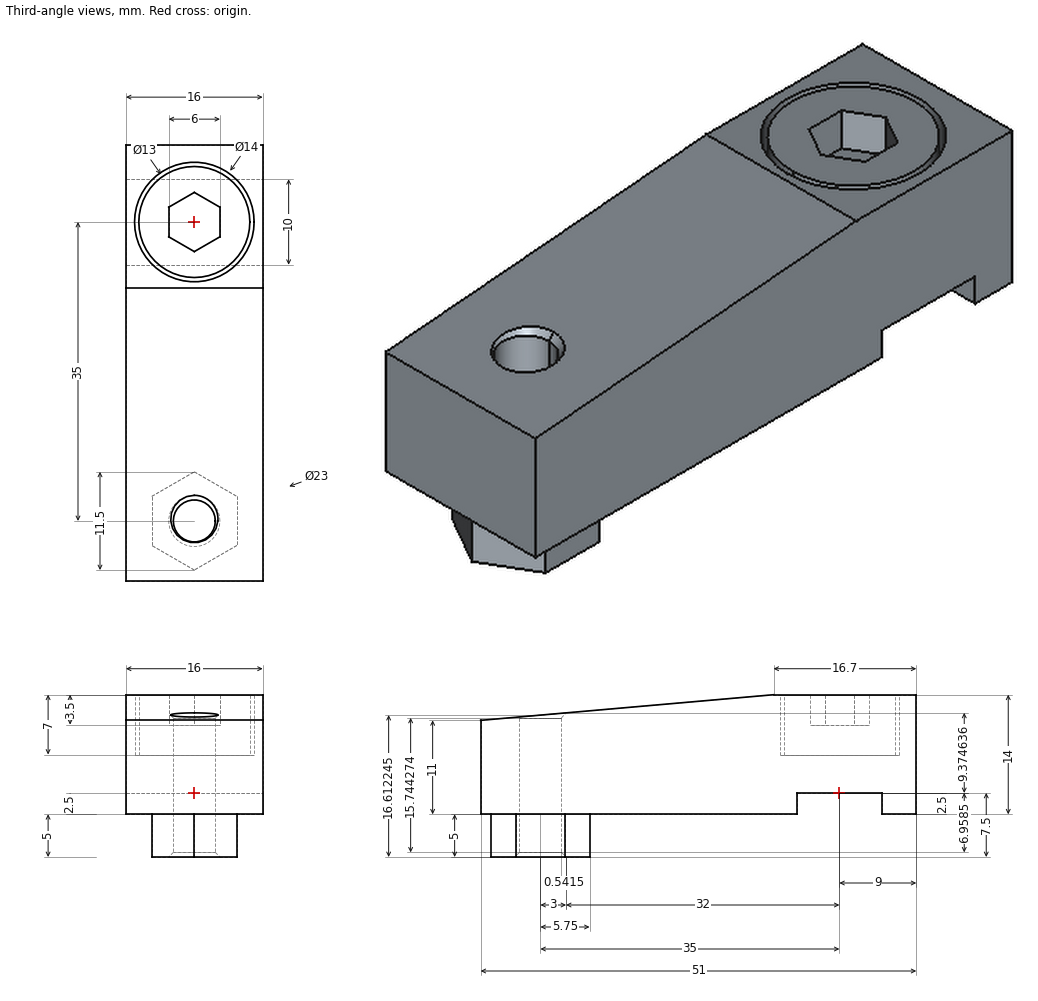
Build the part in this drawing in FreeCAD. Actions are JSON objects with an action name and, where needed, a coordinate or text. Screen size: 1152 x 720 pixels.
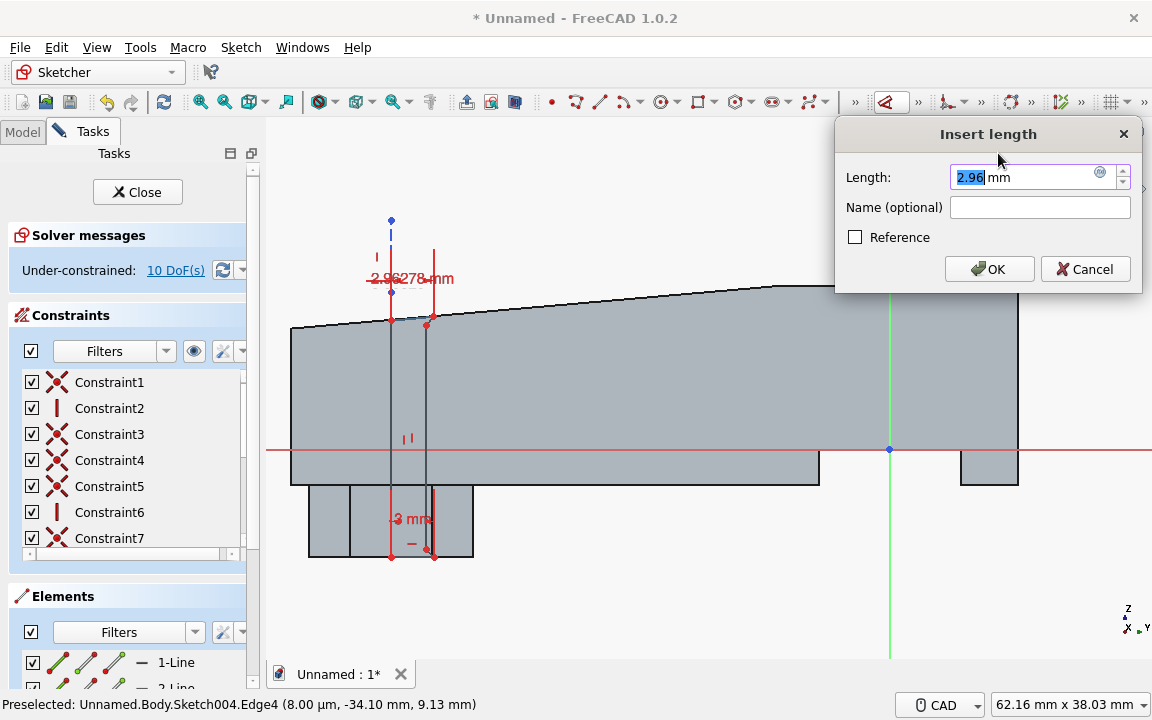
{"action": "type", "text": "3"}
{"action": "key", "text": "Return"}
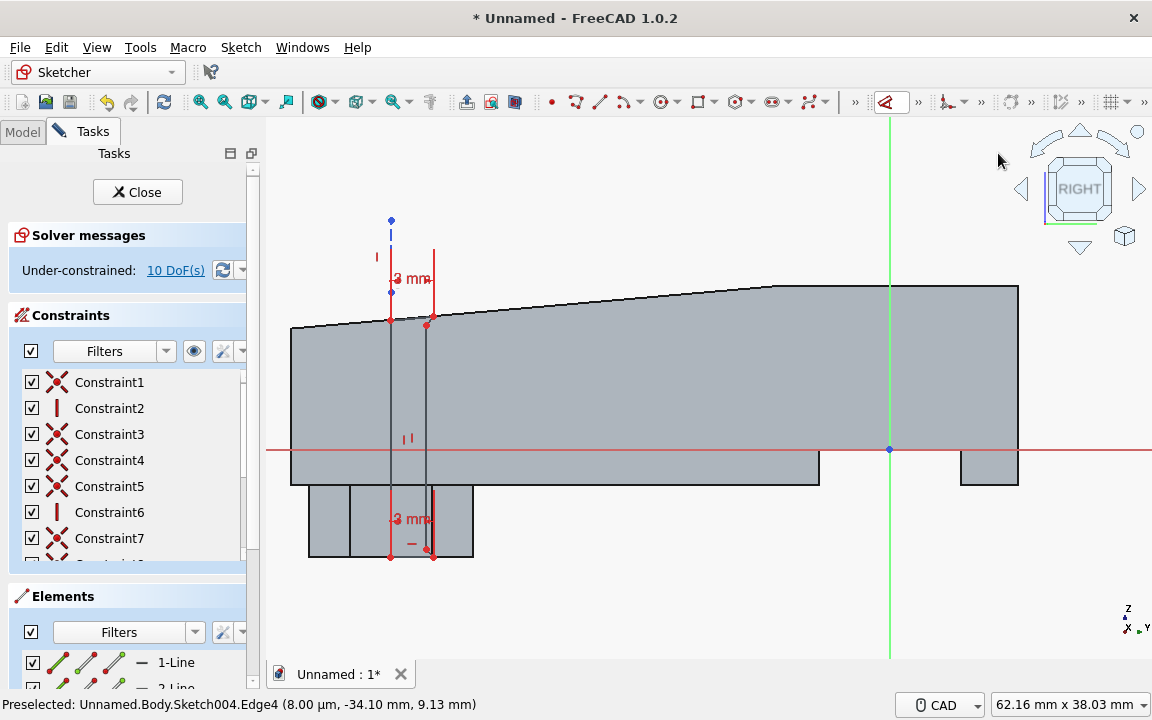
{"action": "left_click", "coordinate": [434, 557]}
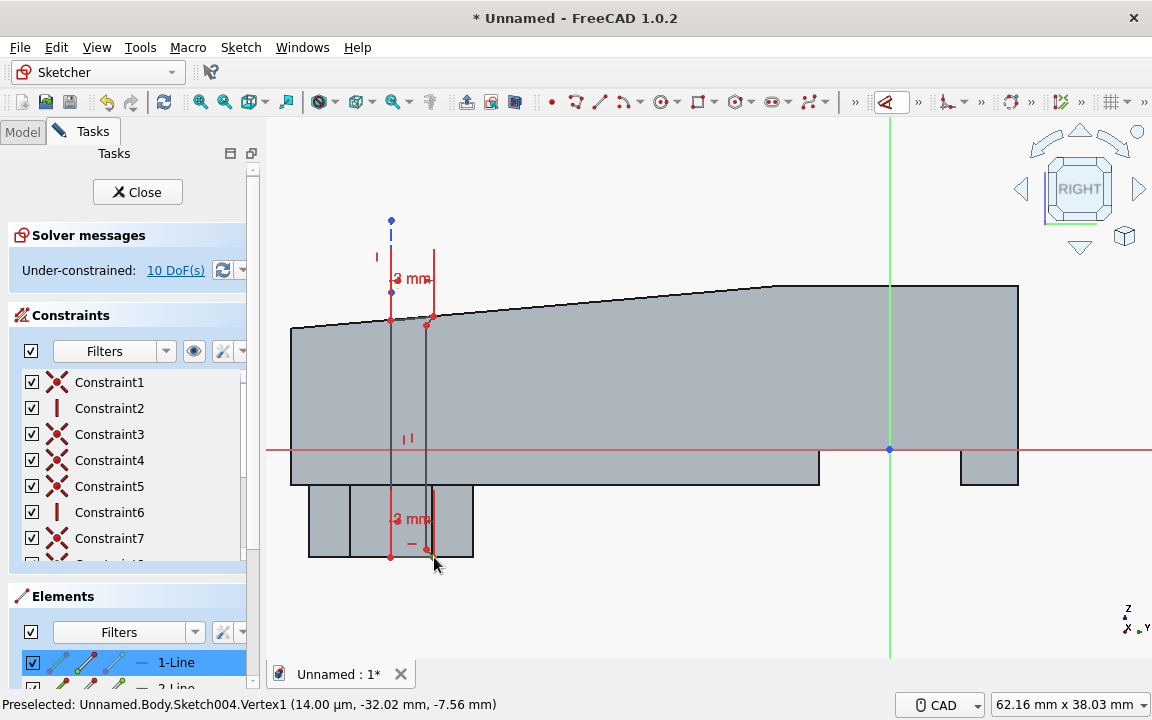
{"action": "key", "text": "l"}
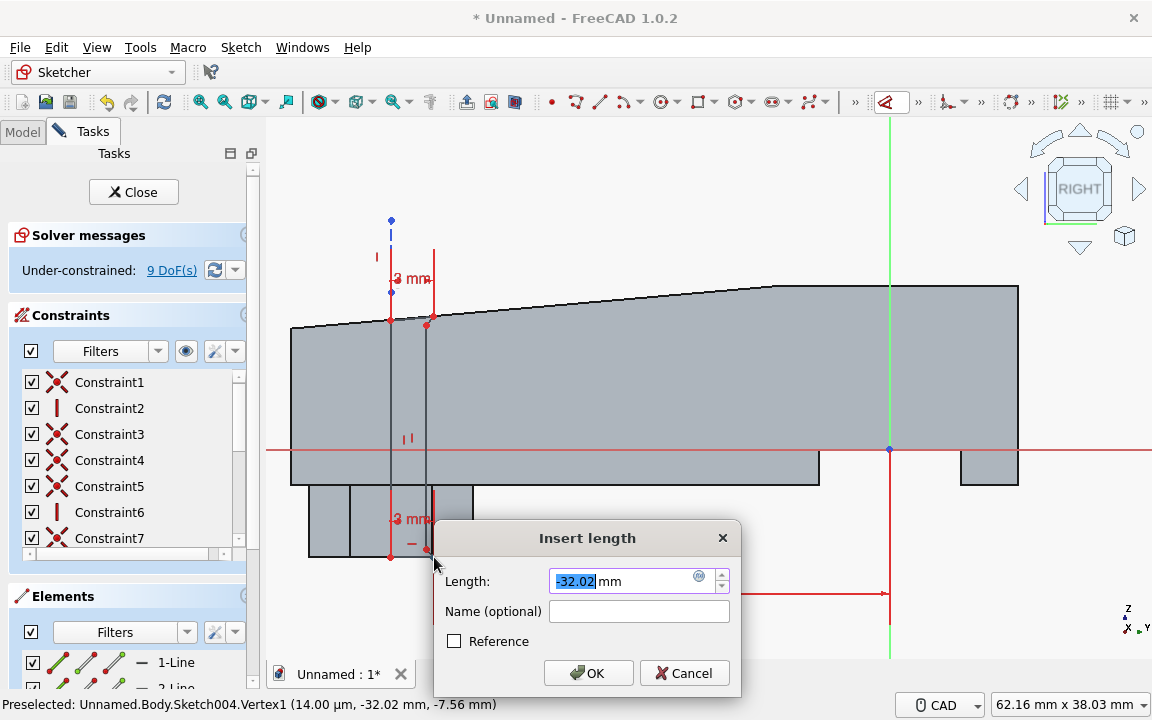
{"action": "type", "text": "-32"}
{"action": "key", "text": "Return"}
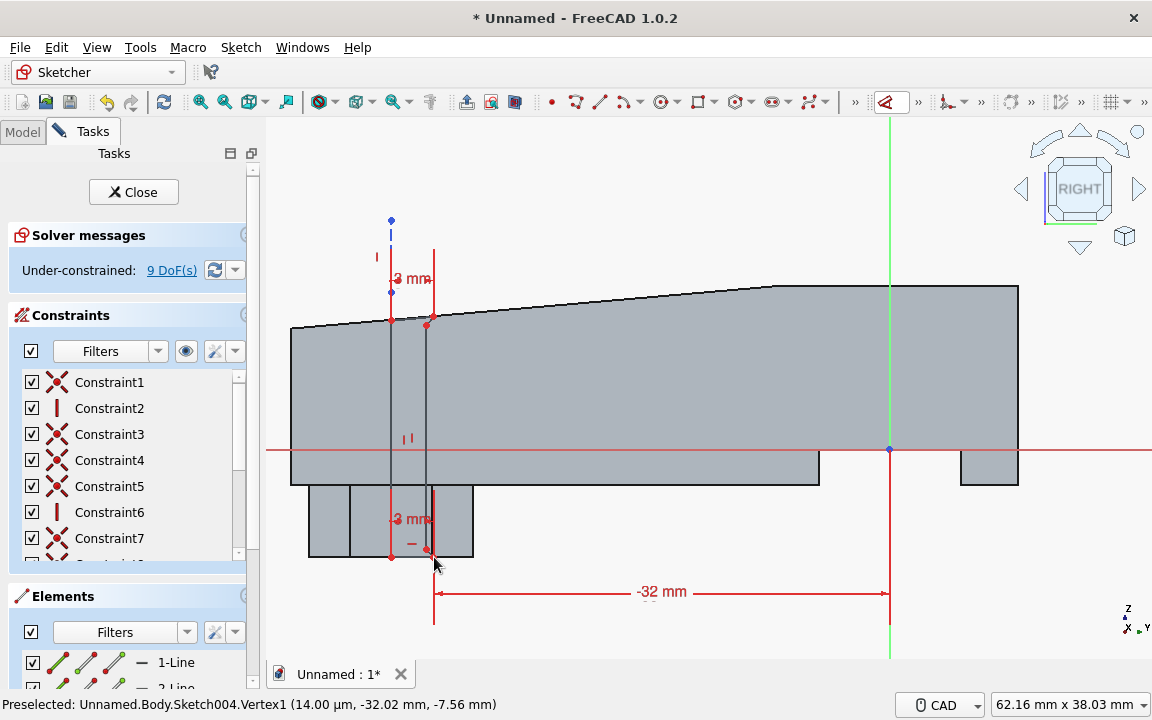
{"action": "left_click", "coordinate": [391, 293]}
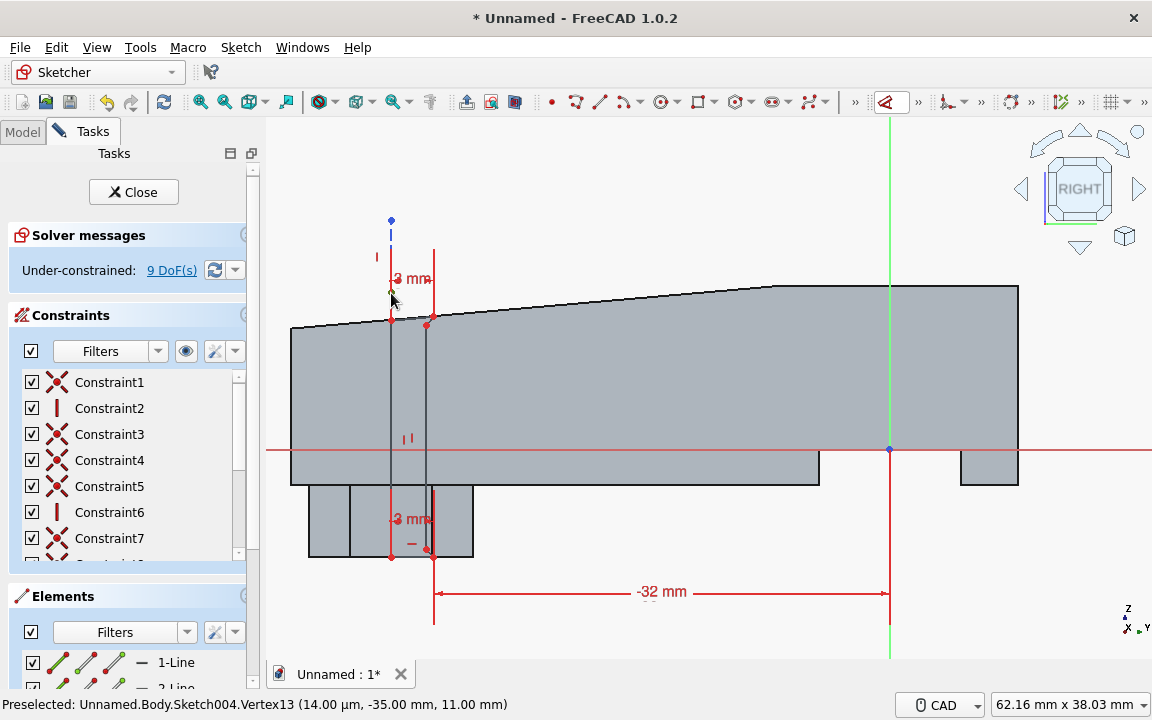
{"action": "key", "text": "l"}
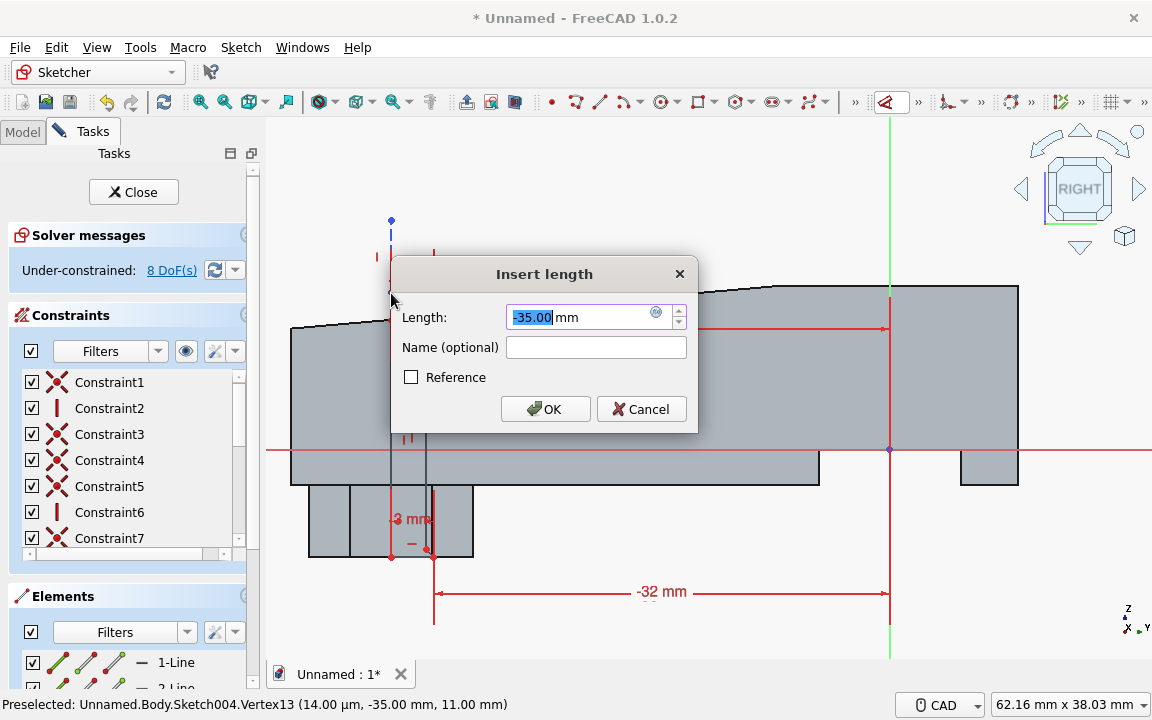
{"action": "type", "text": "-35"}
{"action": "key", "text": "Return"}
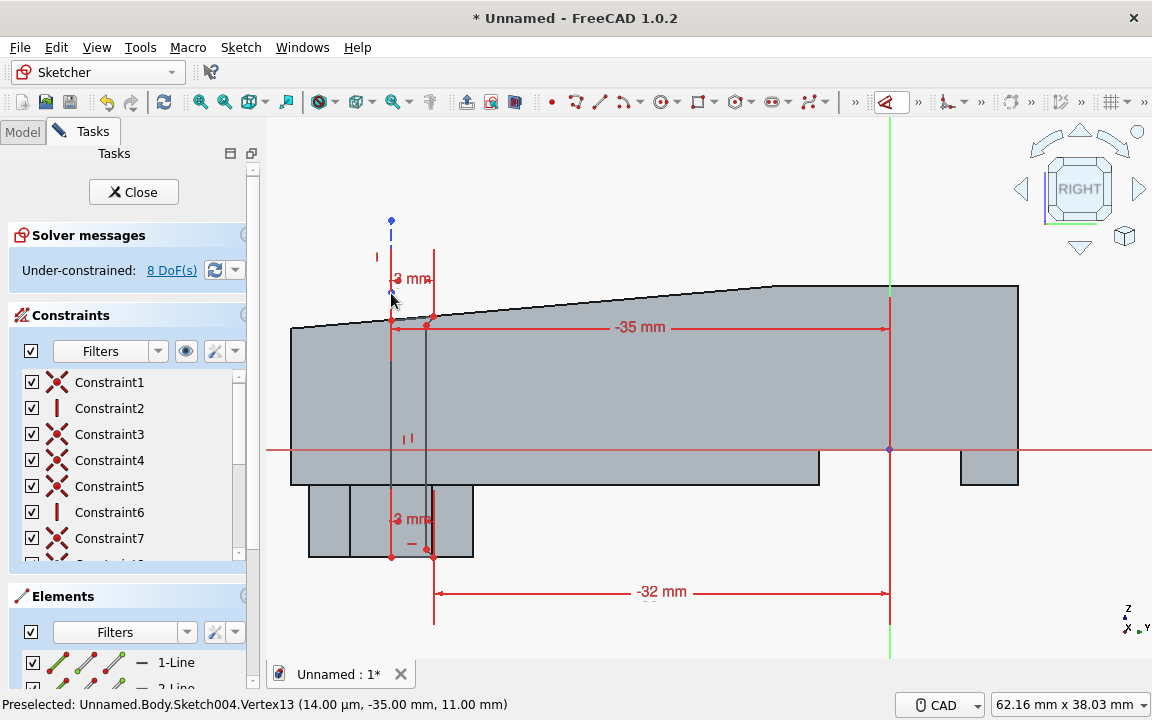
{"action": "left_click", "coordinate": [434, 557]}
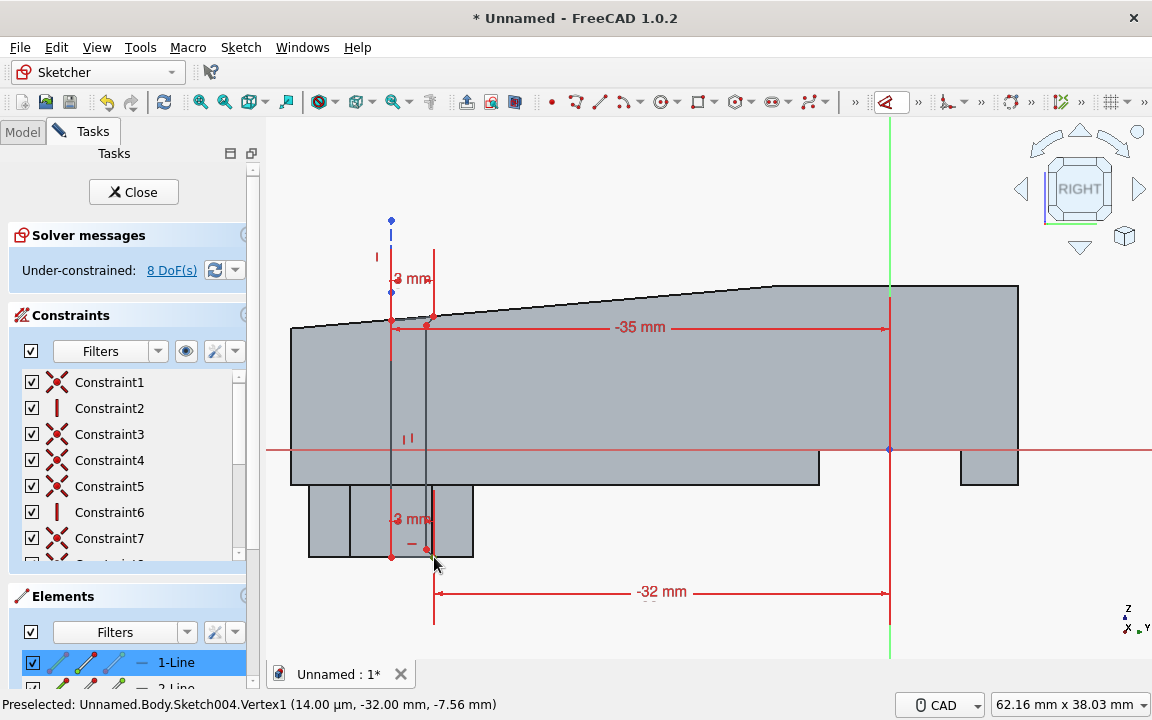
{"action": "key", "text": "i"}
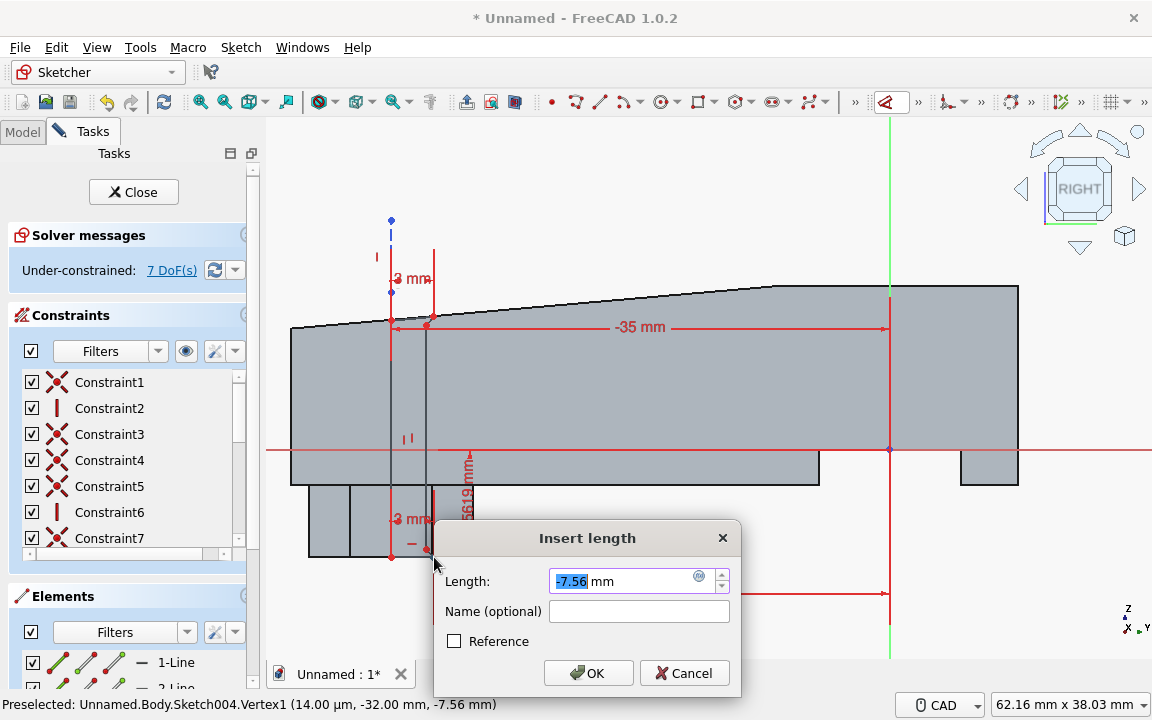
{"action": "type", "text": "-7.5"}
{"action": "key", "text": "Return"}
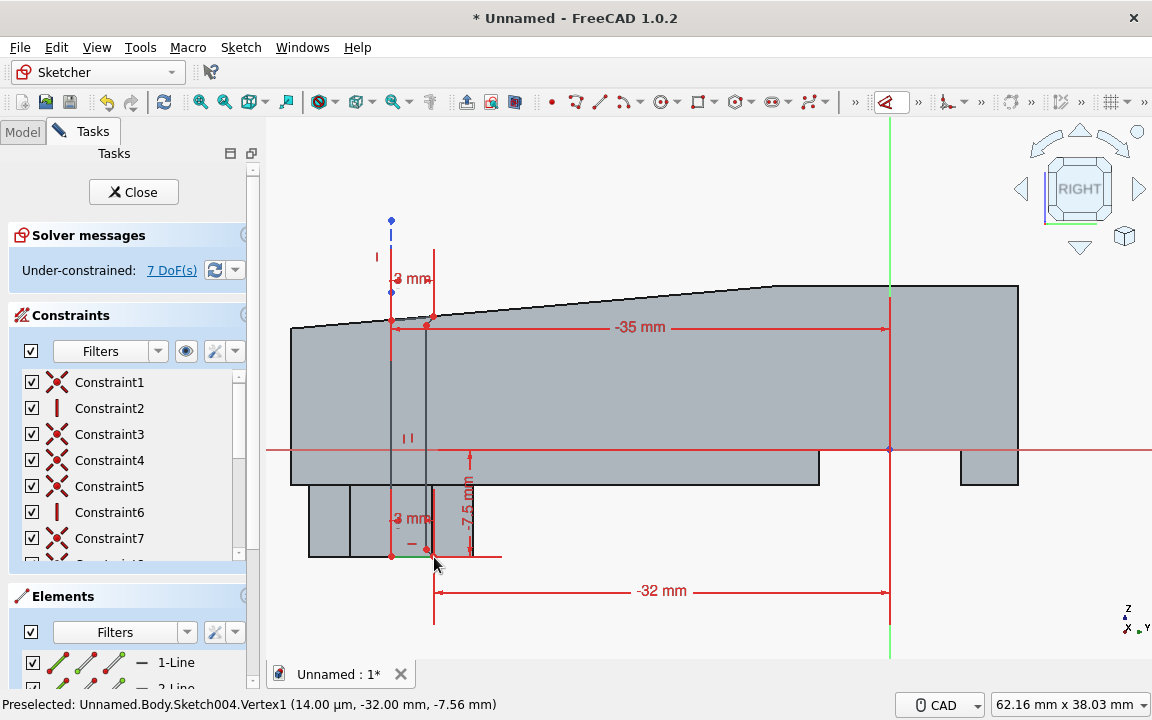
{"action": "left_click", "coordinate": [426, 549]}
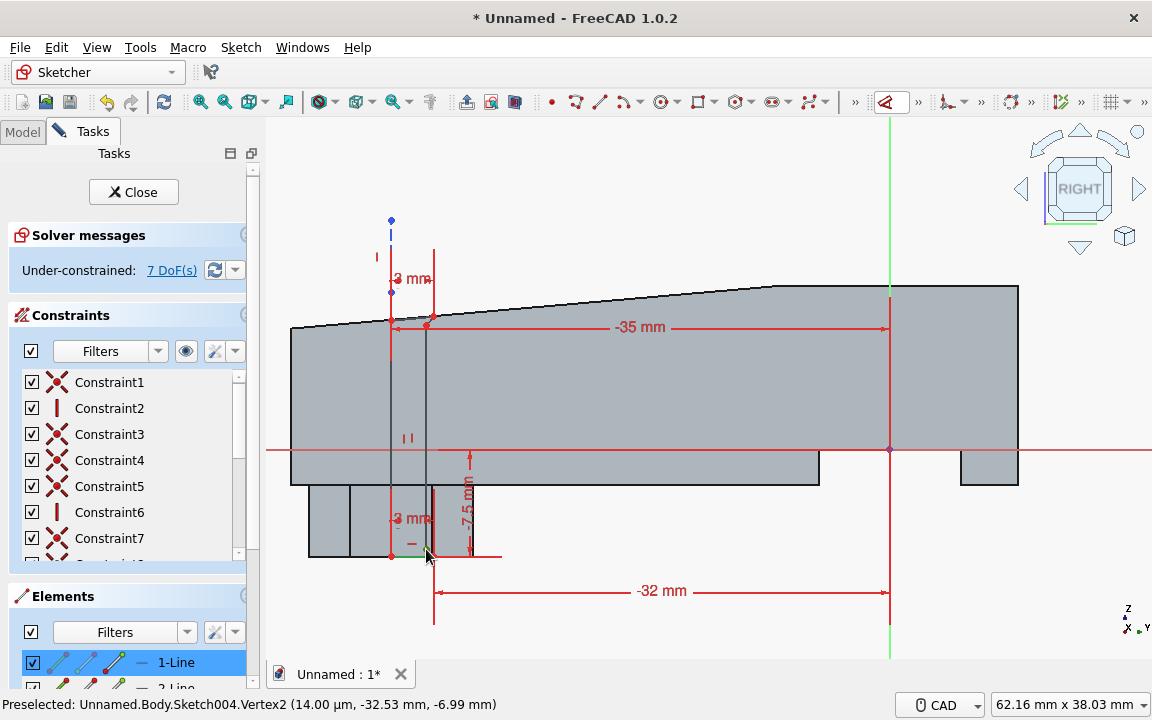
{"action": "left_click", "coordinate": [904, 102]}